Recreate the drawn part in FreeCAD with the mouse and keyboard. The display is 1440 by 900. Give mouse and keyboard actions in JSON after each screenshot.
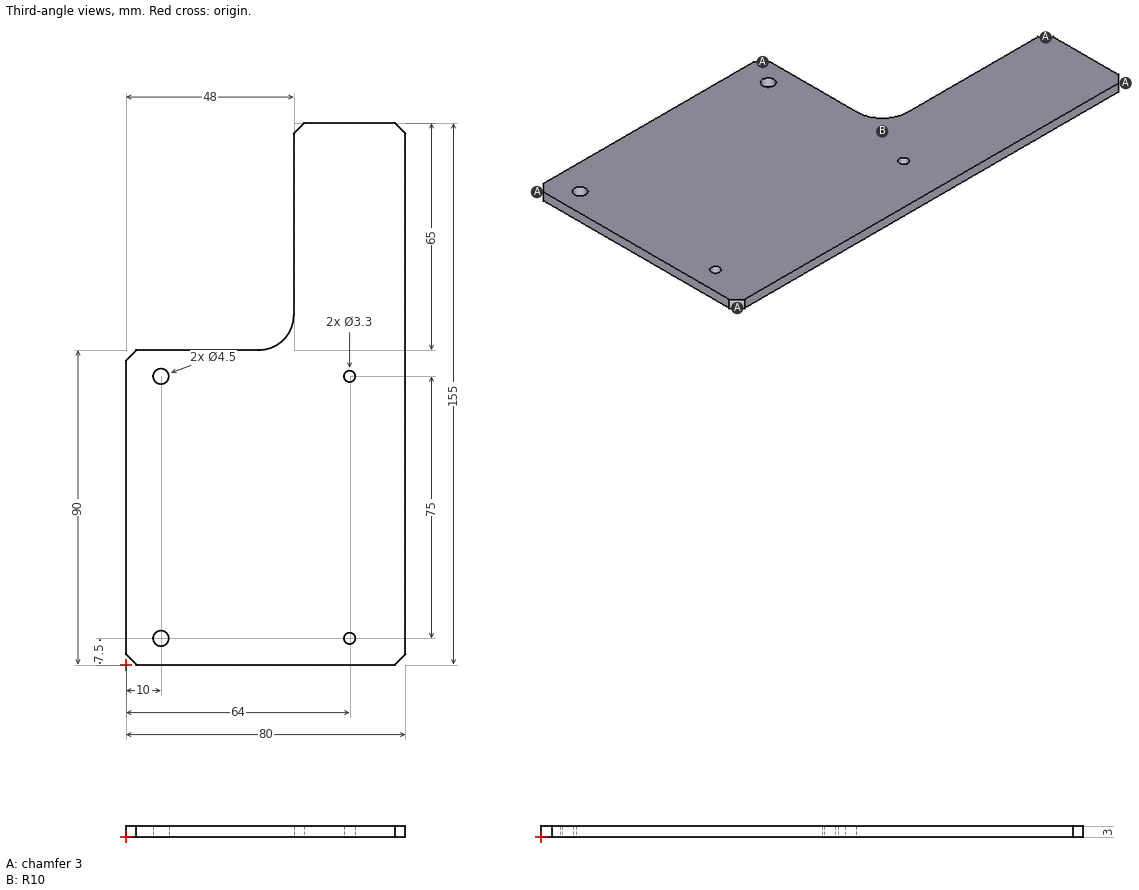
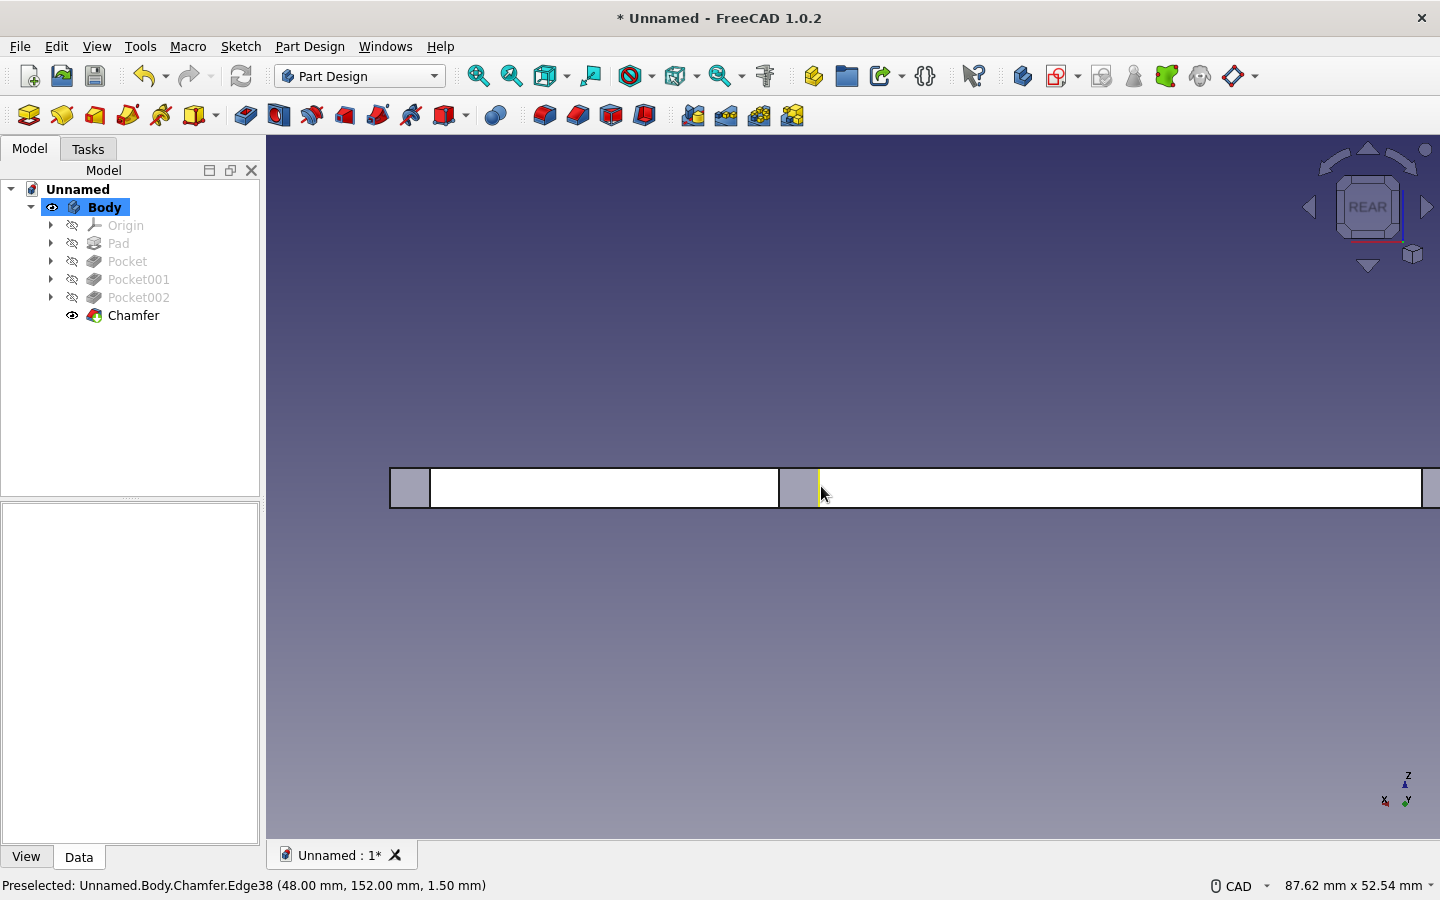
{"action": "key", "text": "v f"}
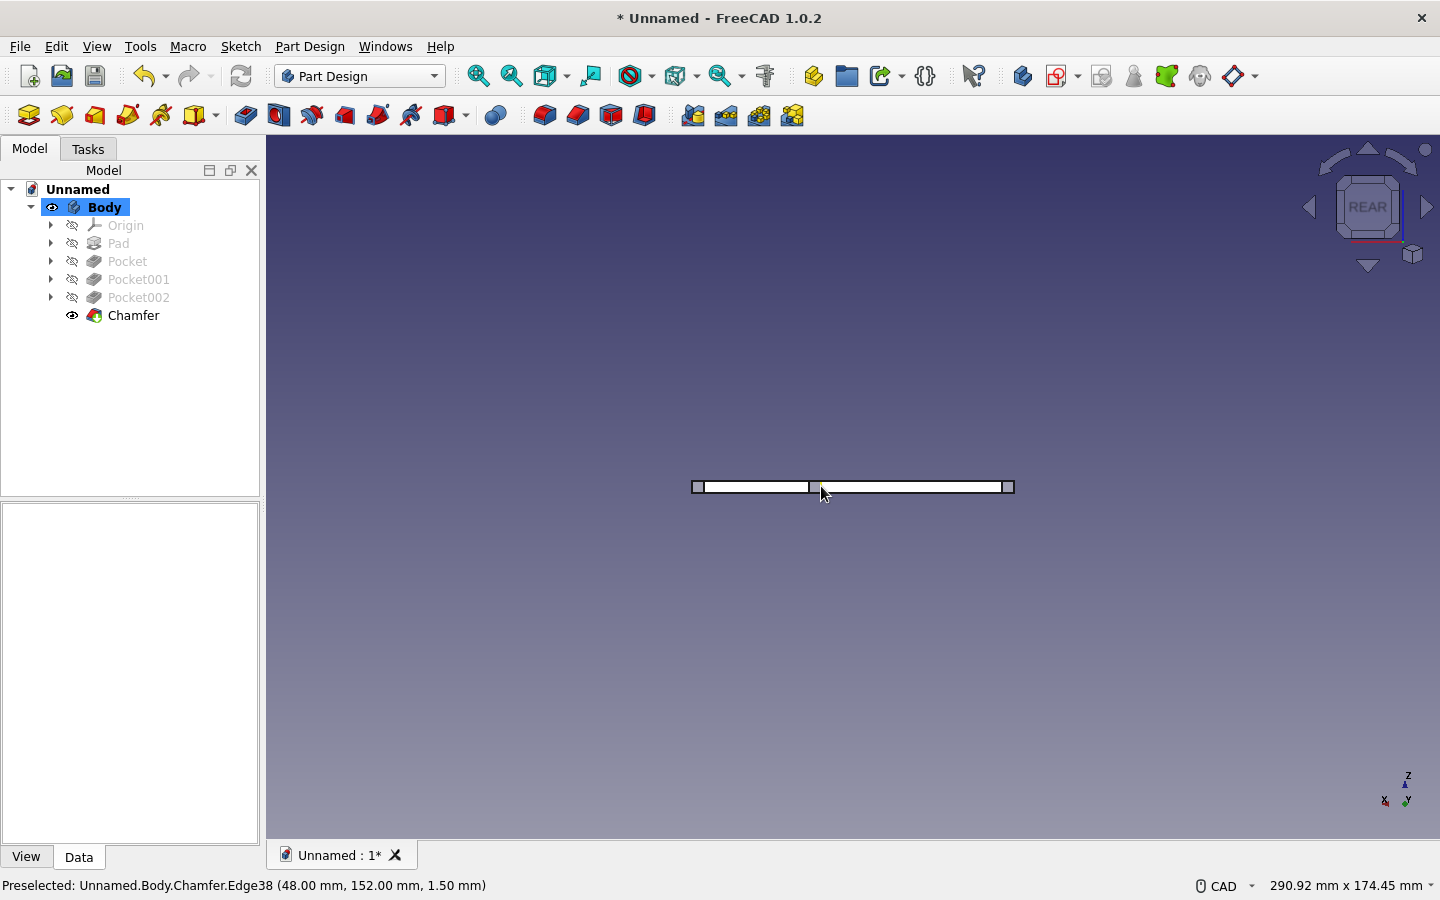
{"action": "key", "text": "0"}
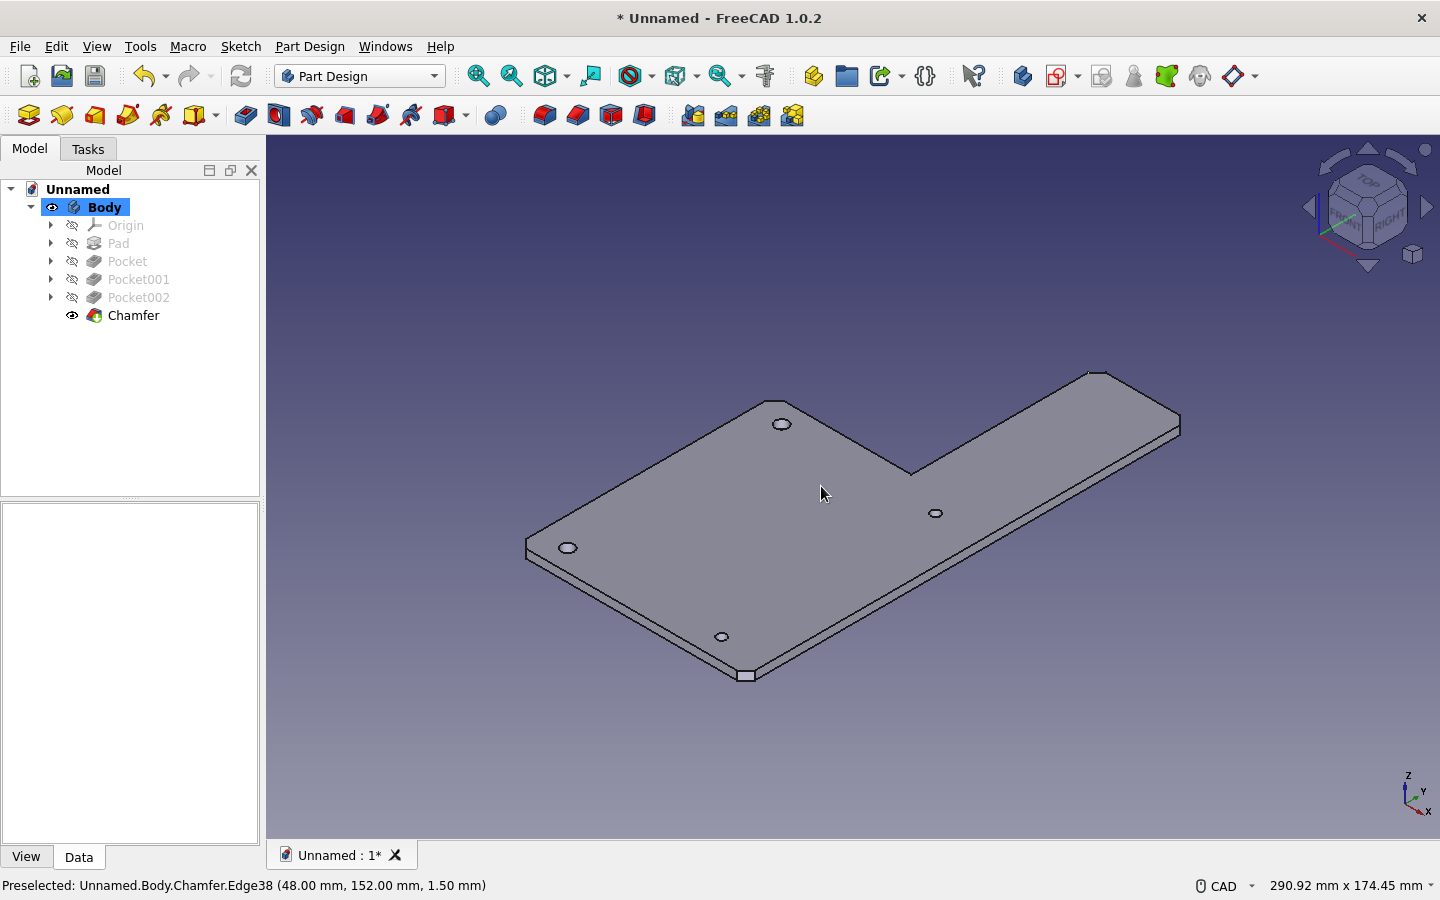
{"action": "scroll", "coordinate": [911, 479], "scroll_direction": "up", "scroll_amount": 6}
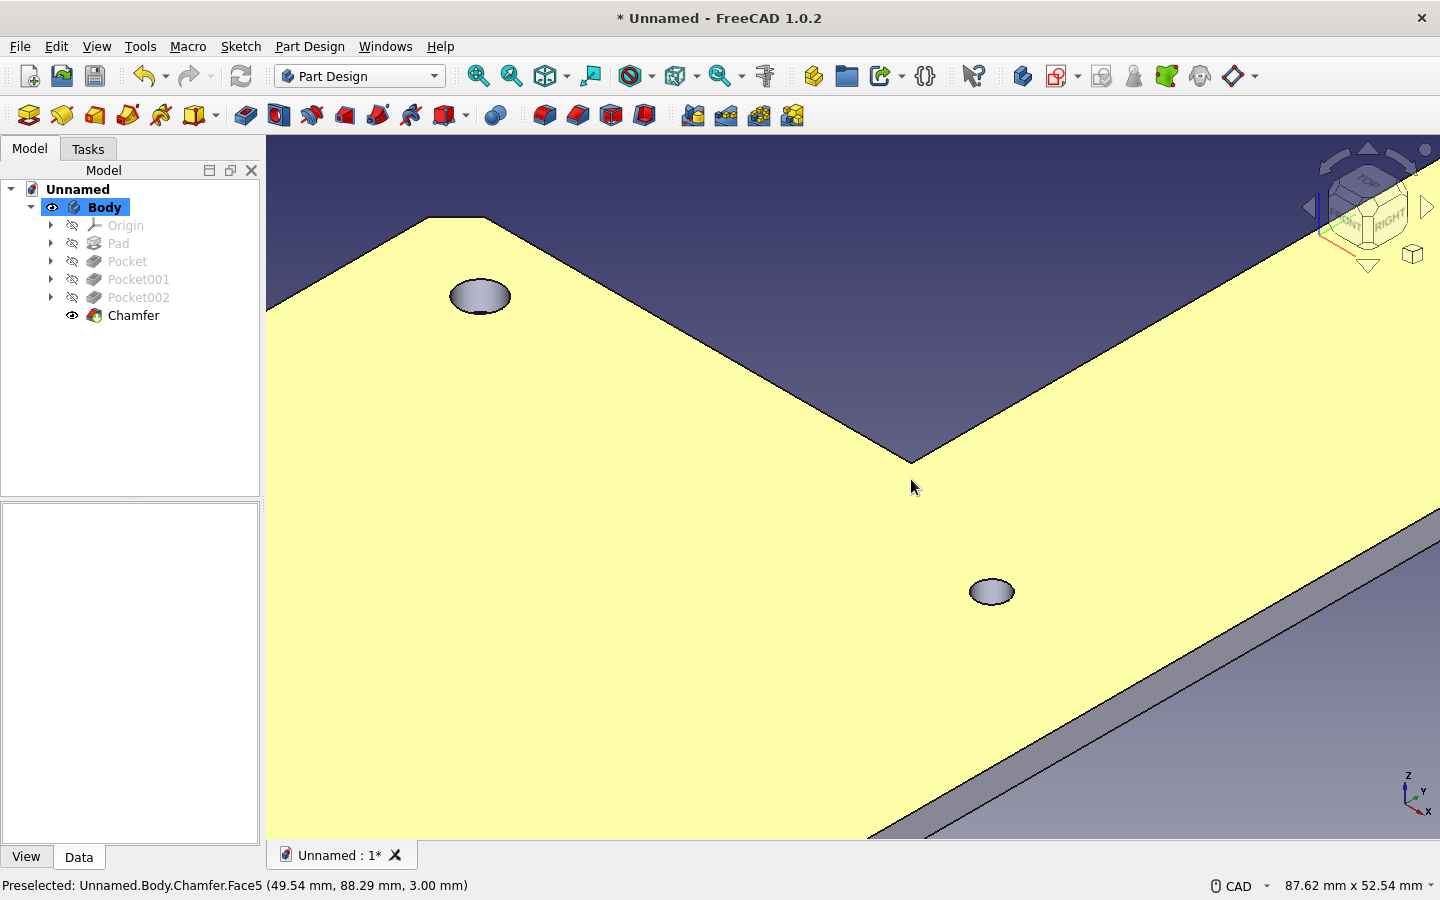
{"action": "key", "text": "v f"}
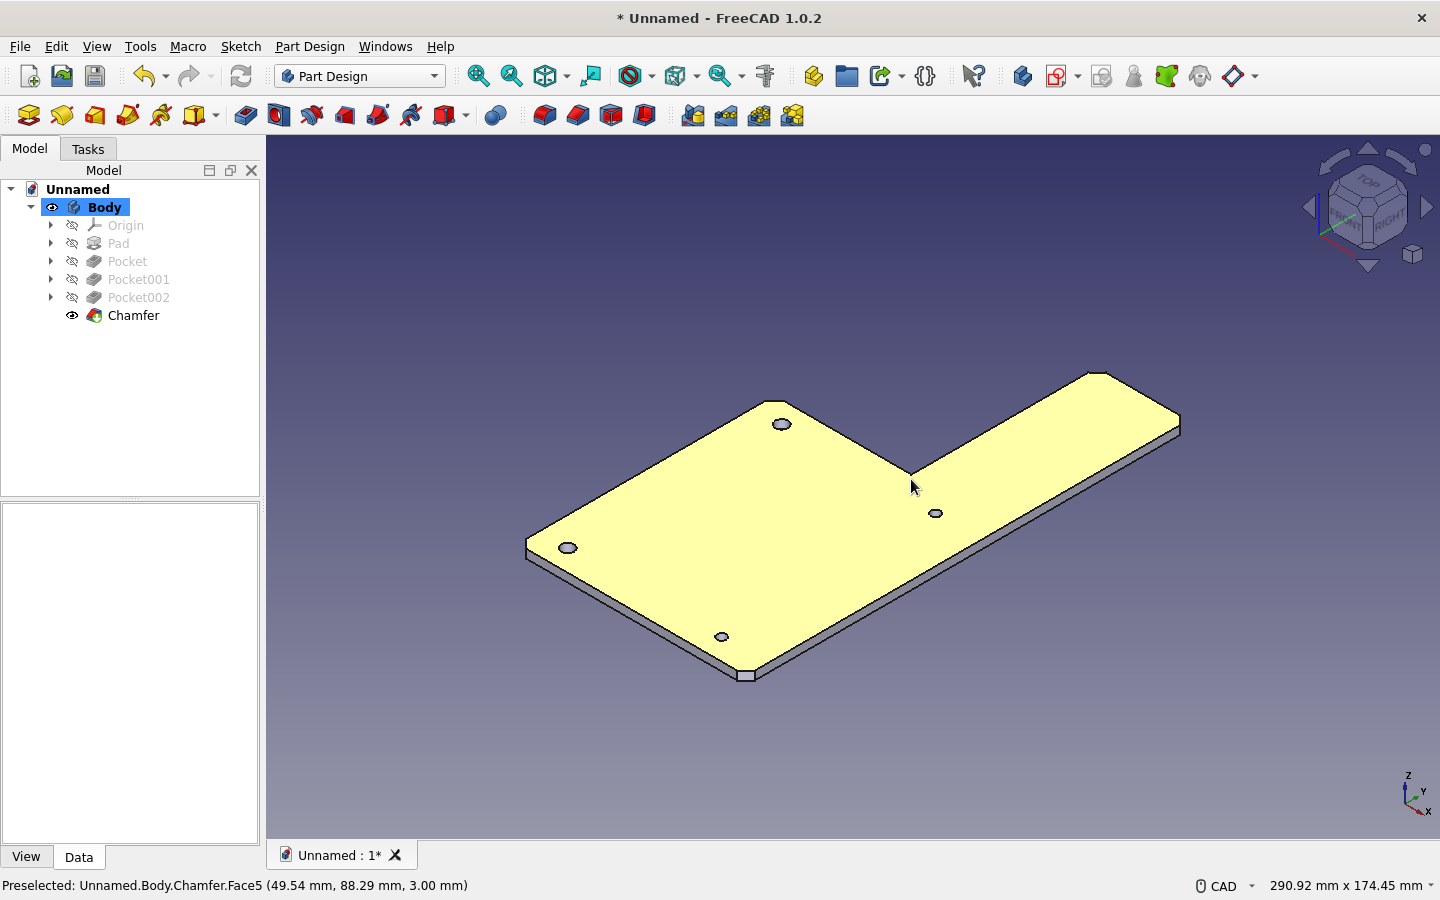
{"action": "key", "text": "2"}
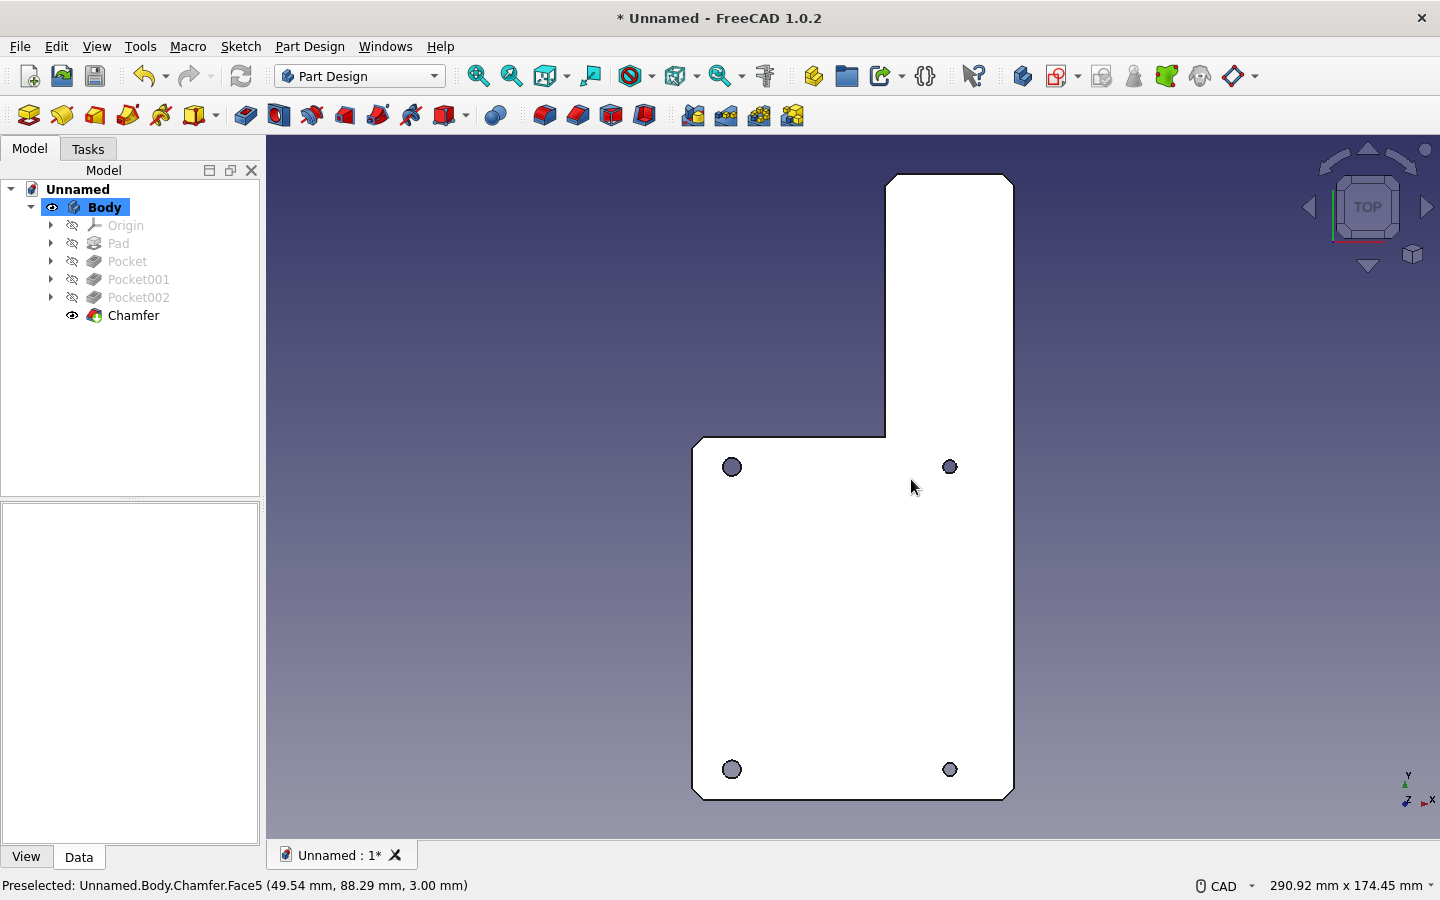
{"action": "scroll", "coordinate": [885, 436], "scroll_direction": "up", "scroll_amount": 6}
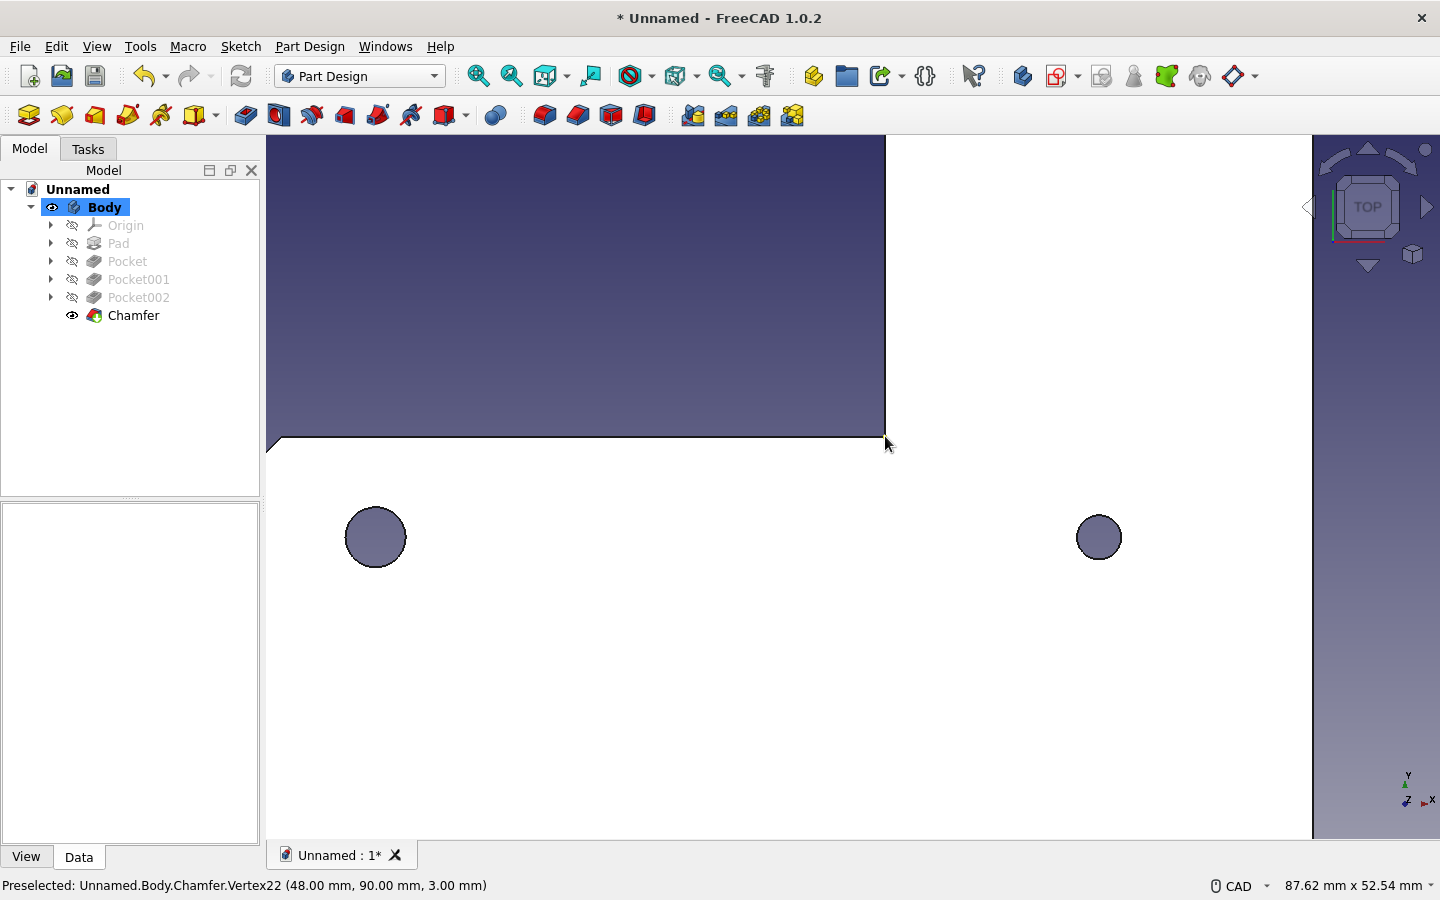
{"action": "key", "text": "v f"}